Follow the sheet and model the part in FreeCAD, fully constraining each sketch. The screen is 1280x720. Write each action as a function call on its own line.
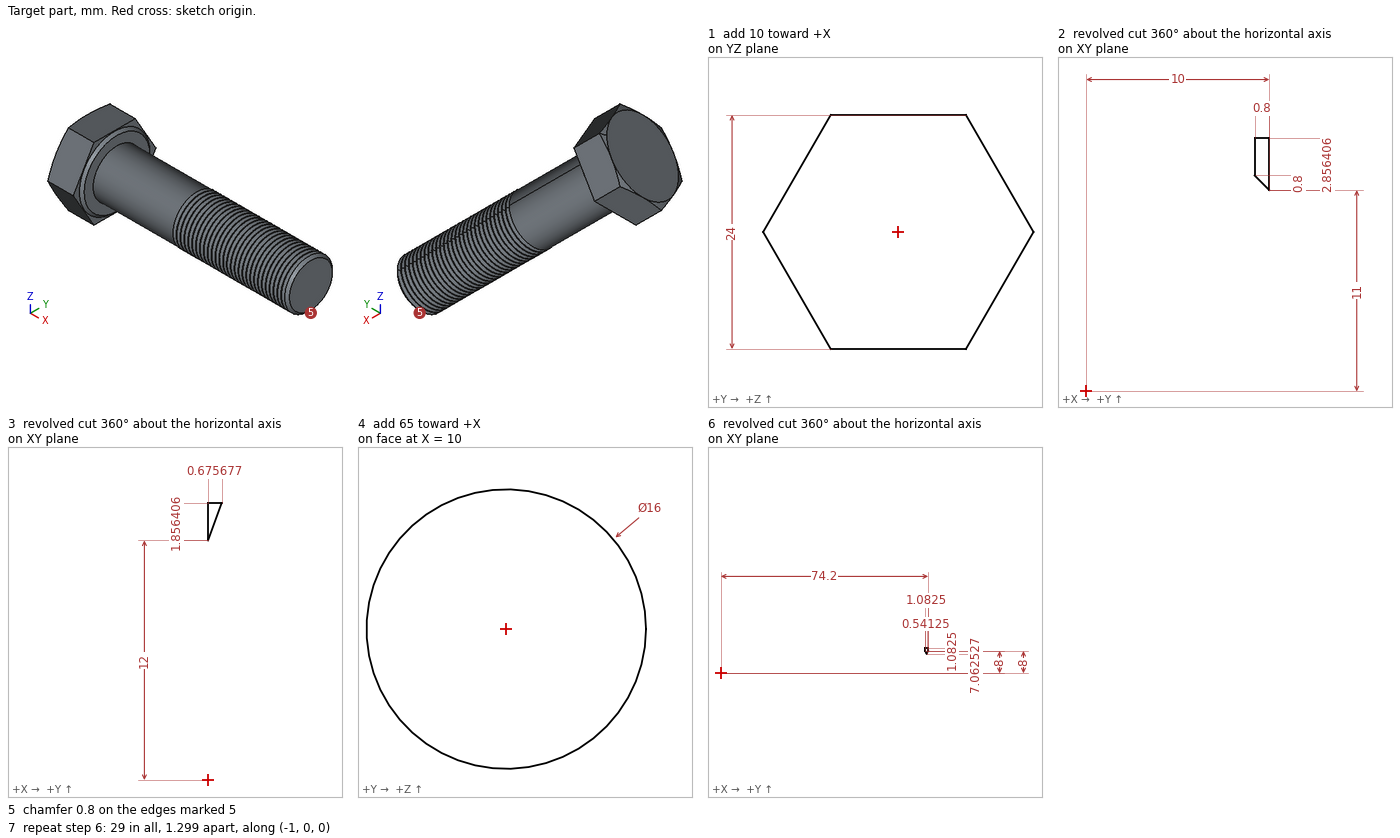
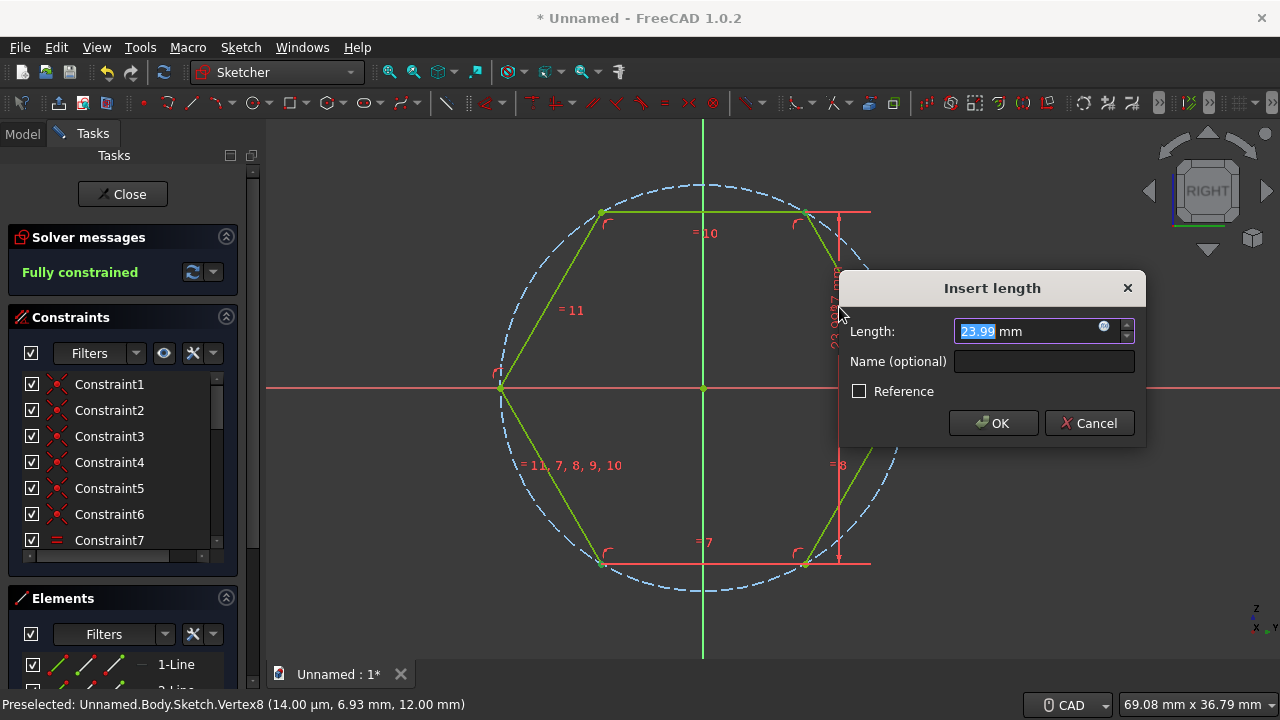
text(24)
key(Return)
key(Escape)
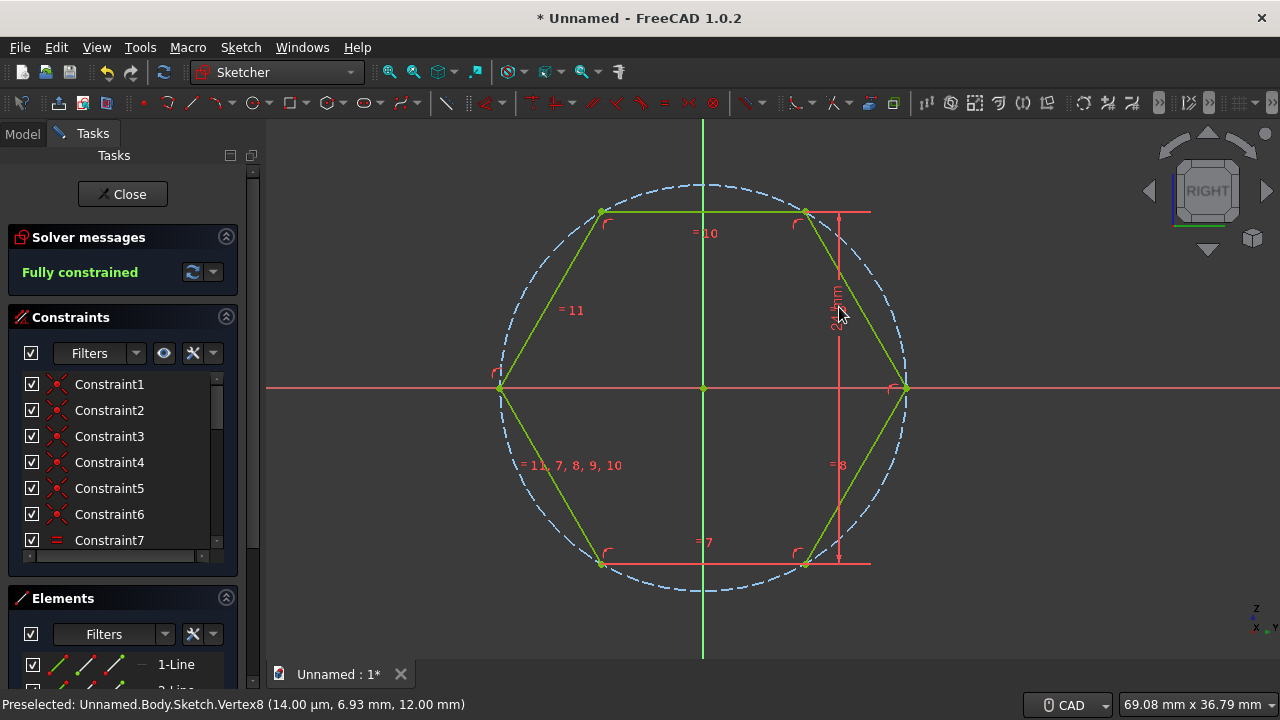
click(123, 194)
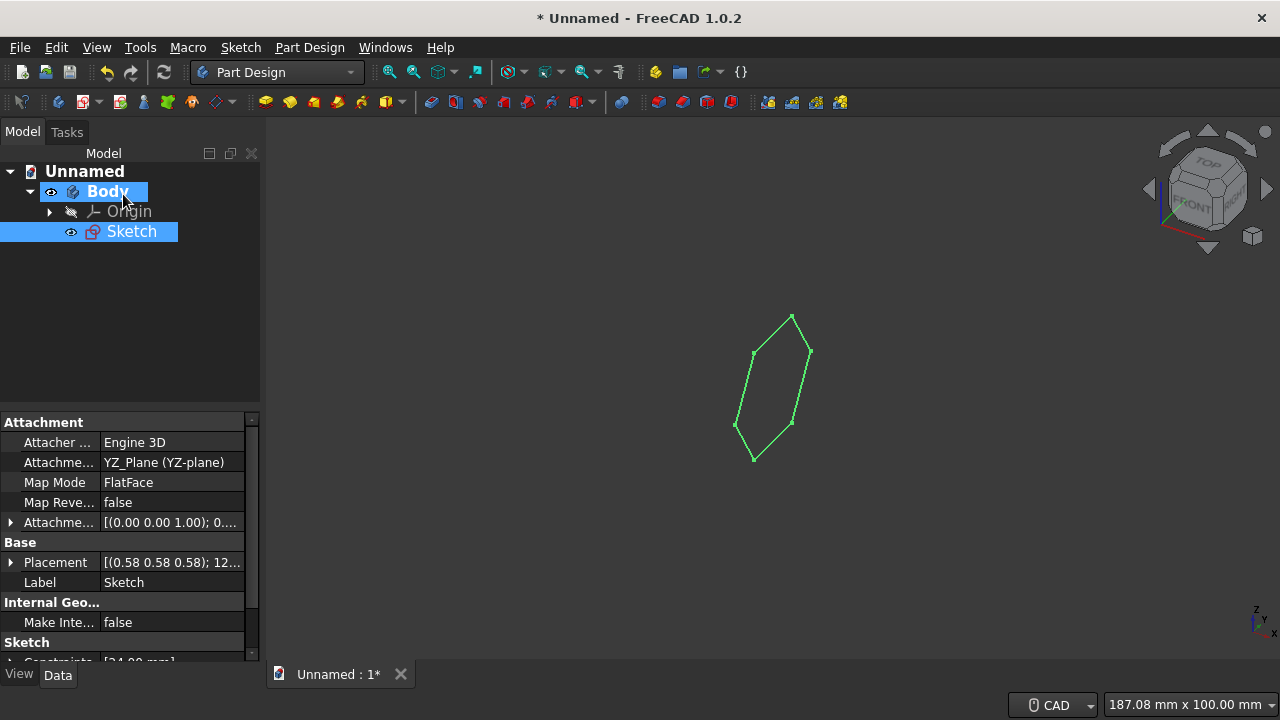
click(266, 102)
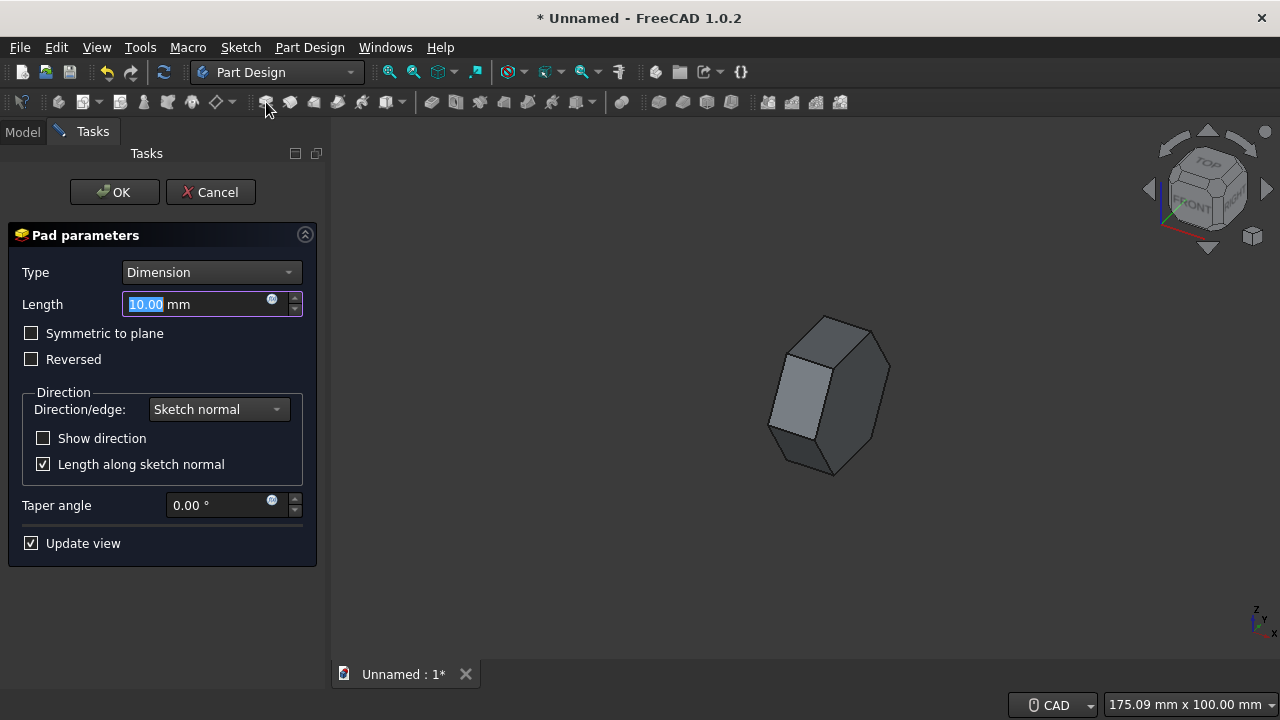
text(10)
key(Tab)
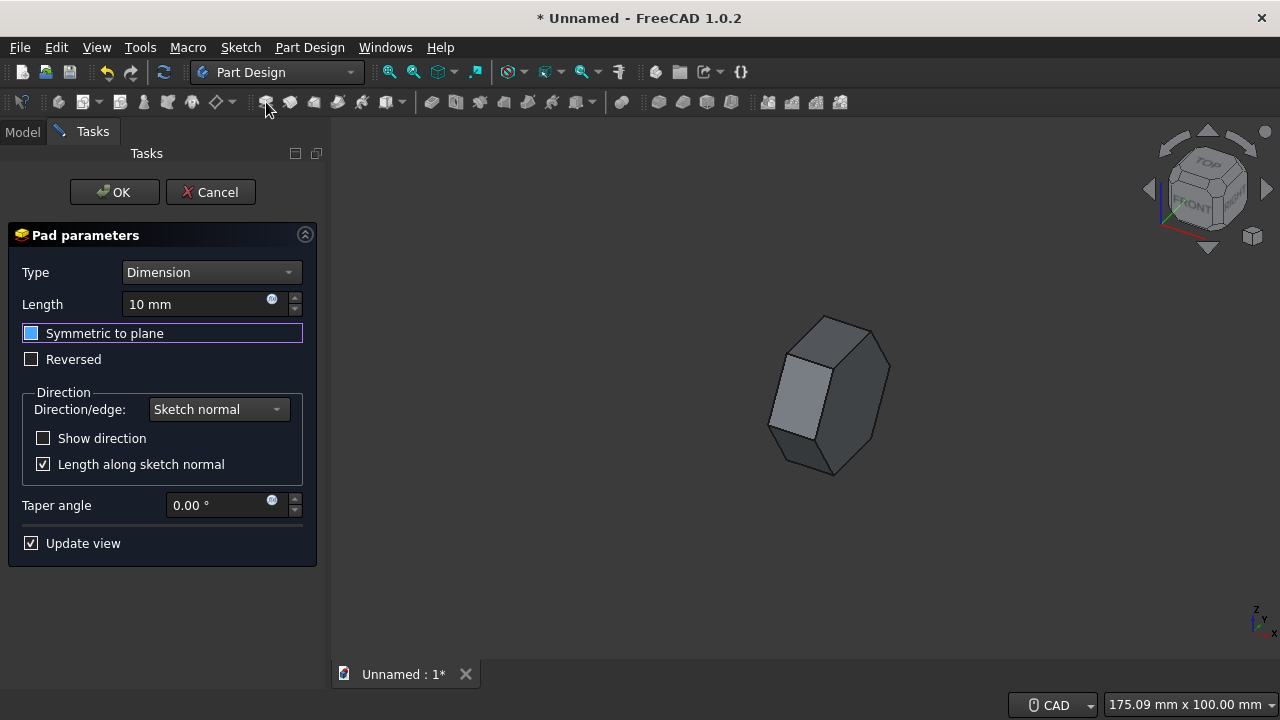
click(115, 192)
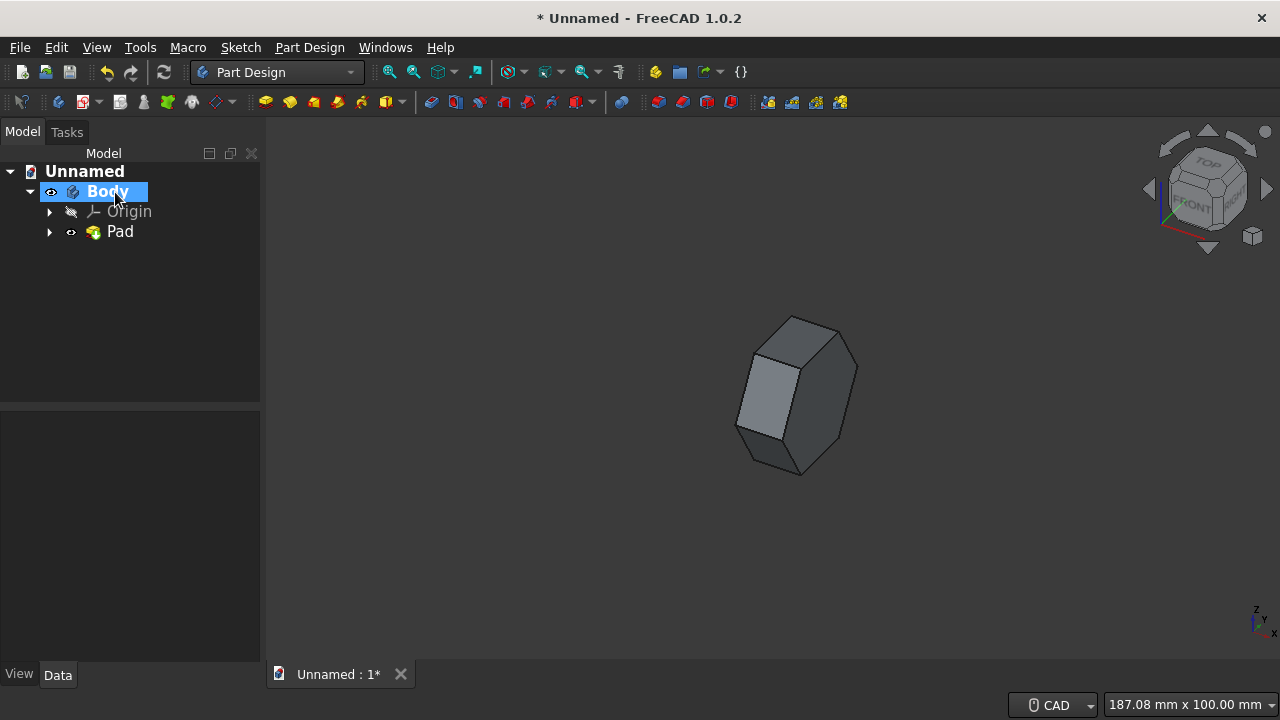
click(390, 72)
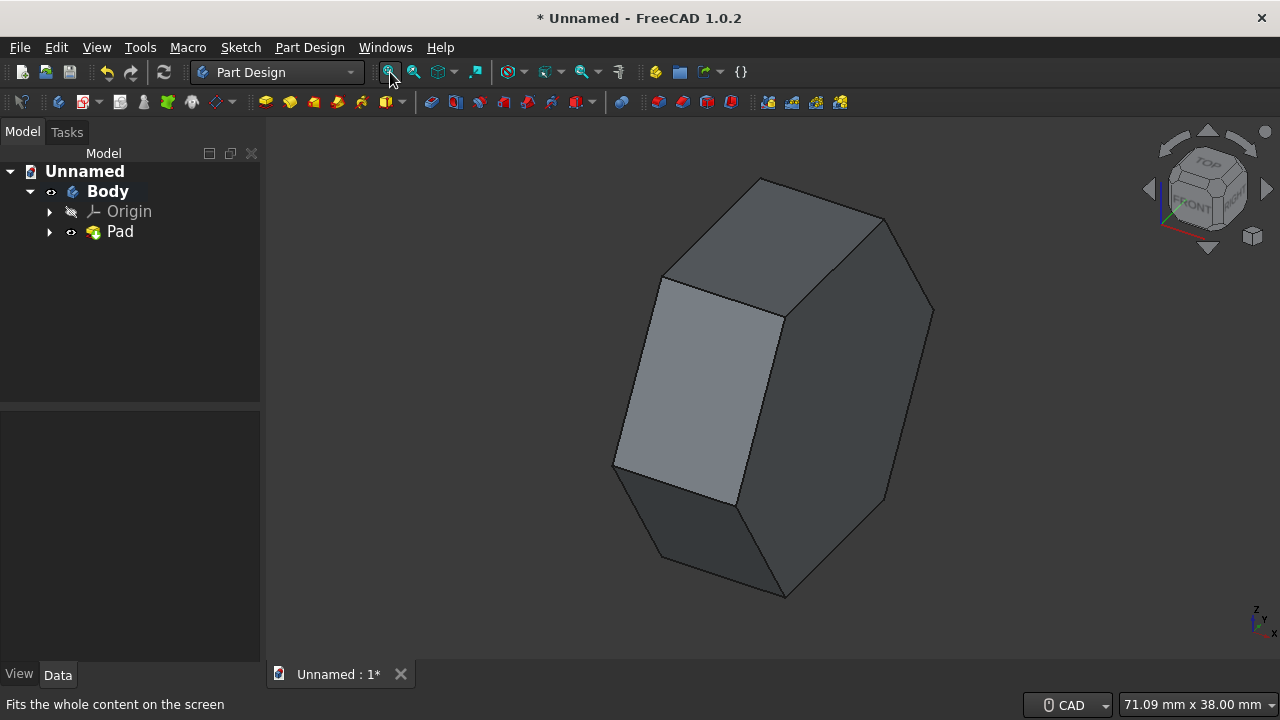
click(84, 102)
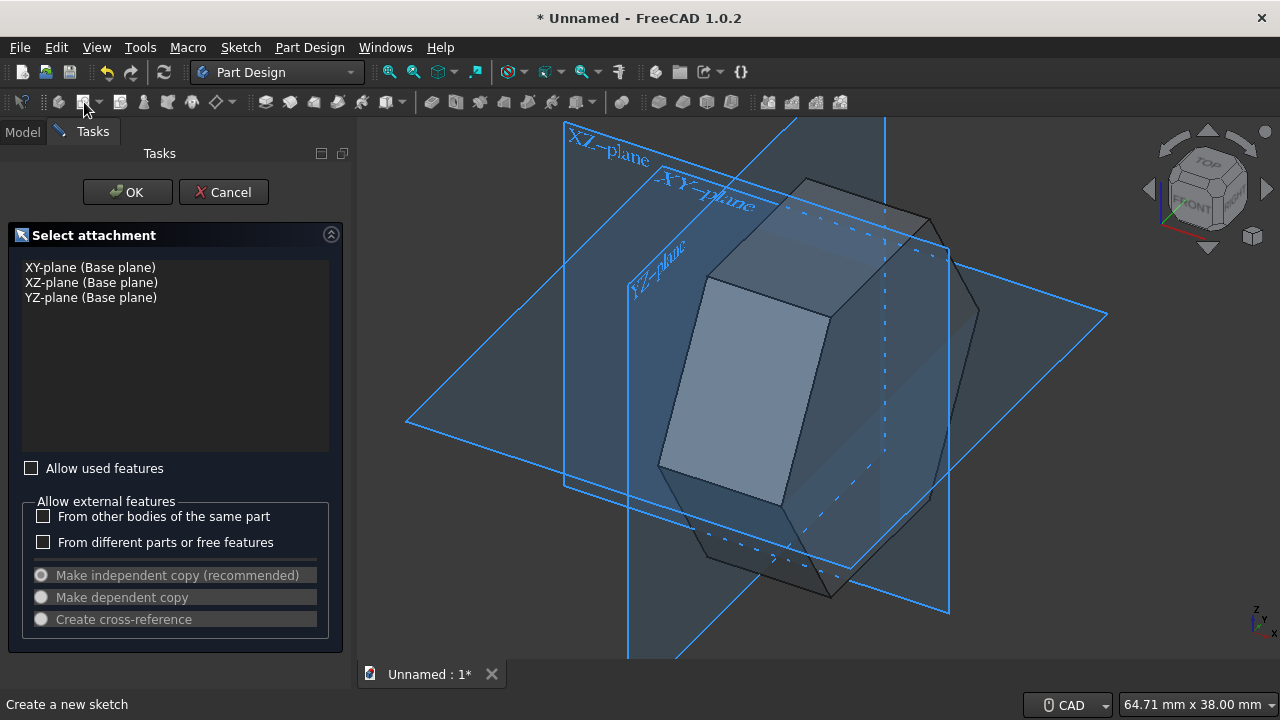
click(82, 268)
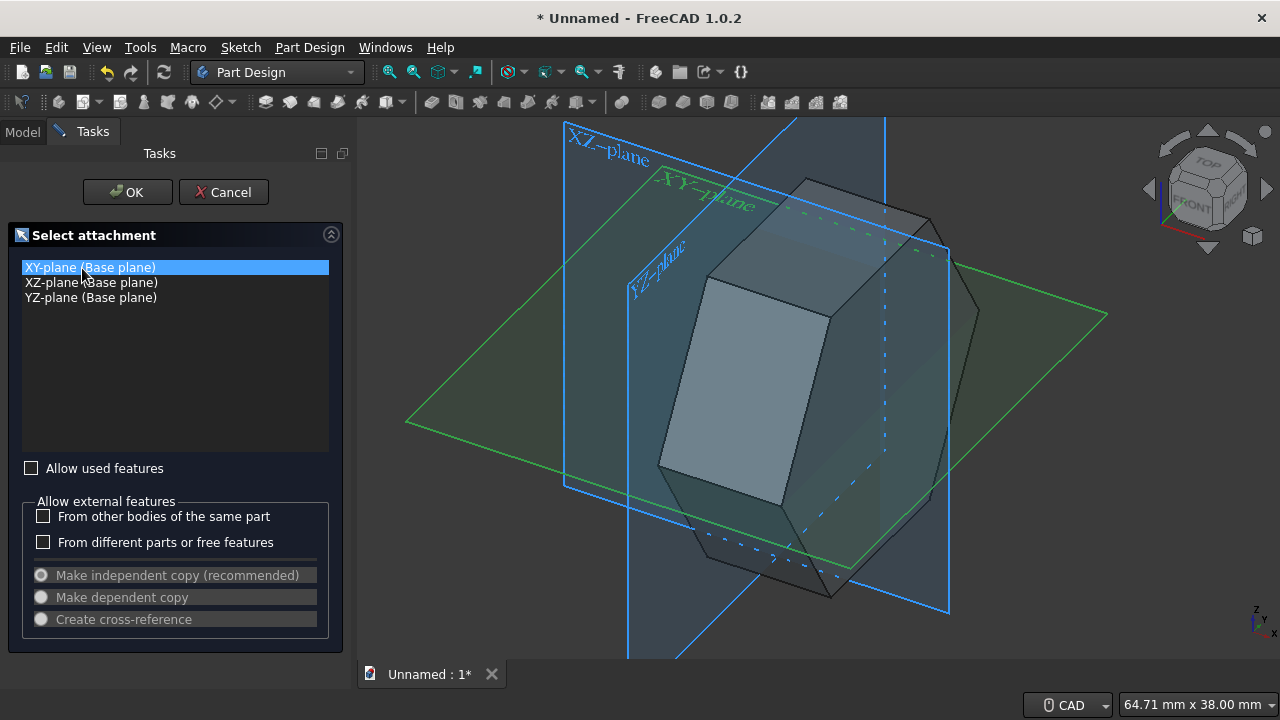
click(128, 192)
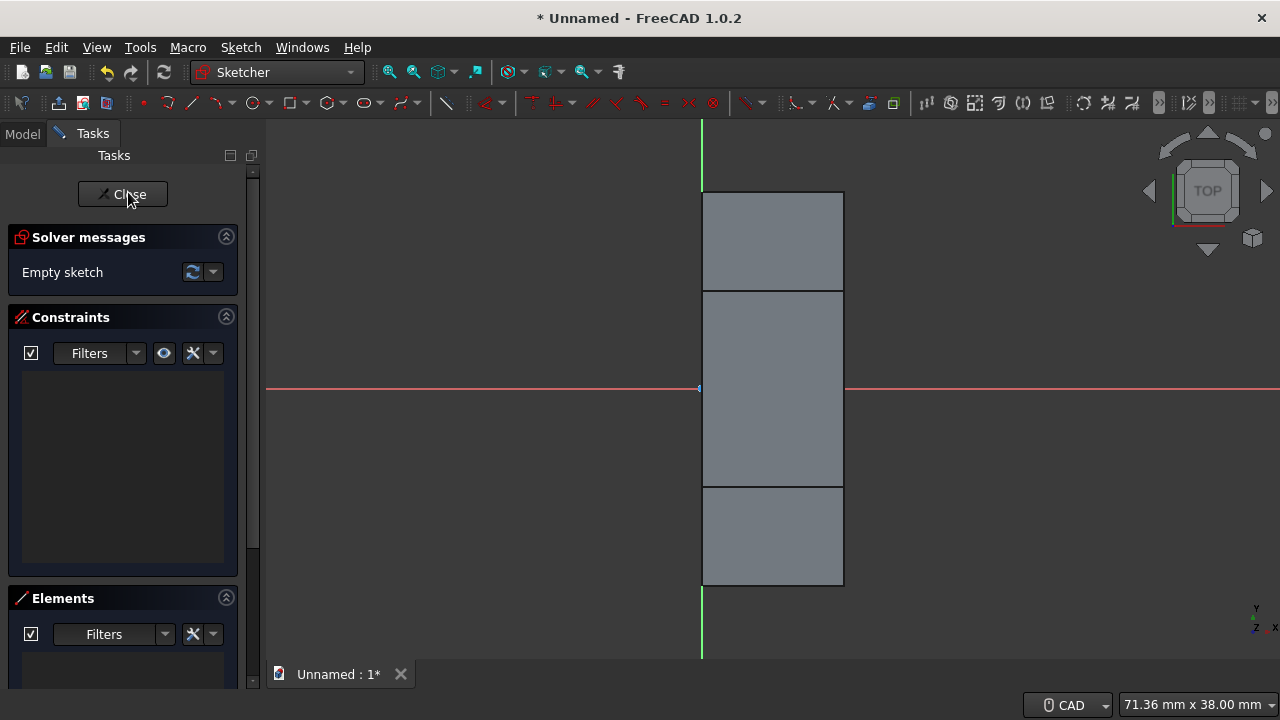
click(108, 104)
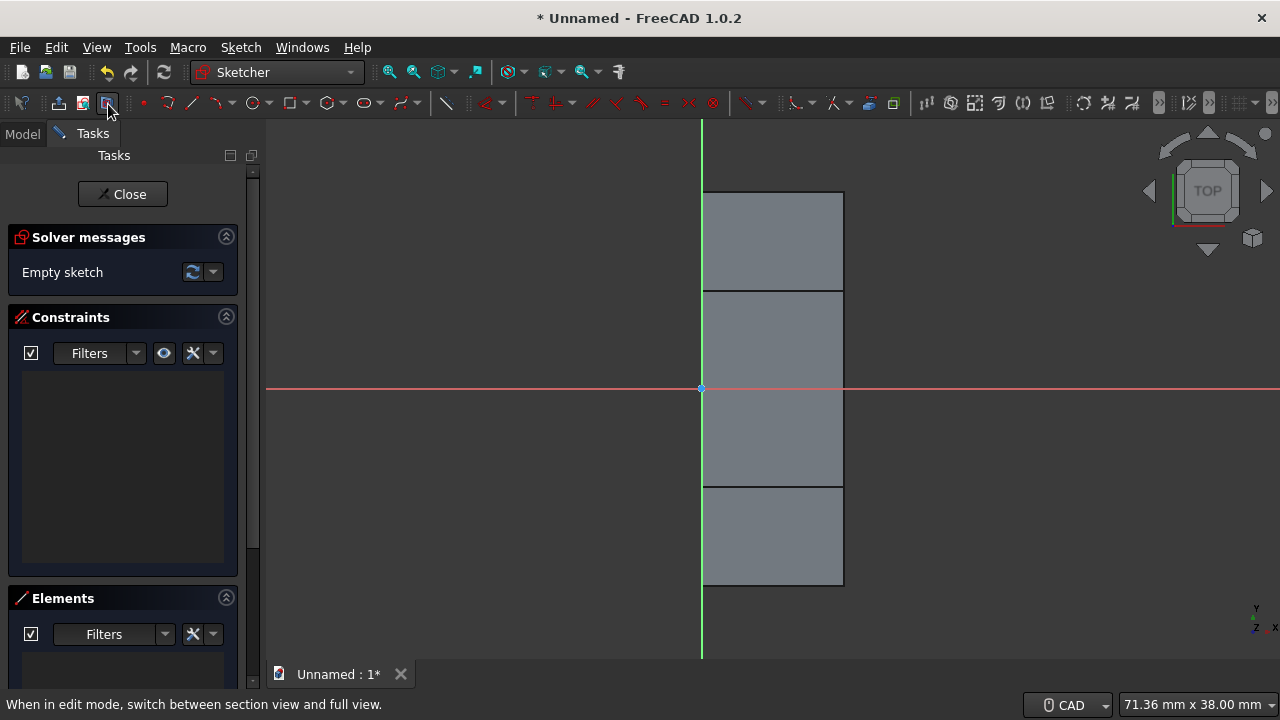
scroll(855, 190, up, 11)